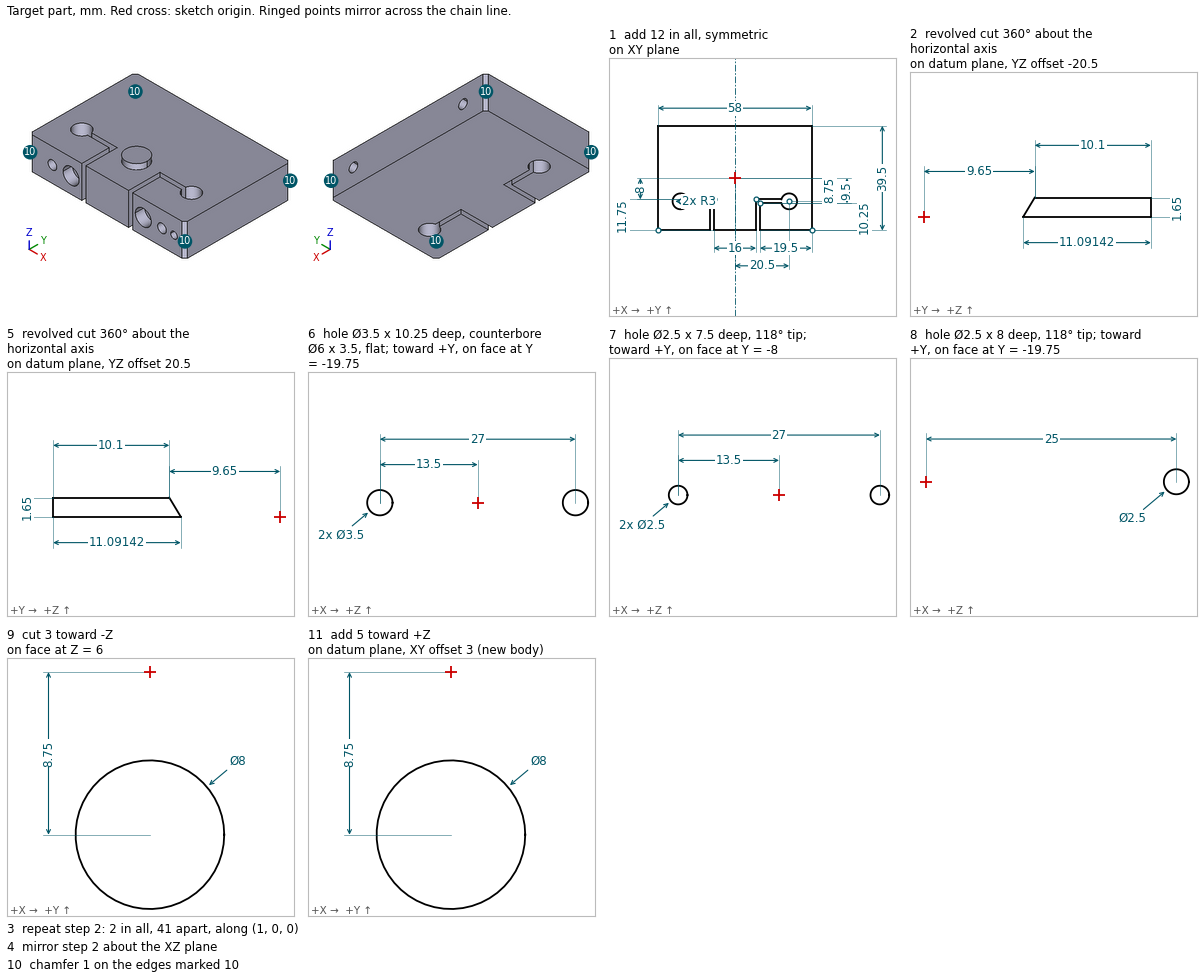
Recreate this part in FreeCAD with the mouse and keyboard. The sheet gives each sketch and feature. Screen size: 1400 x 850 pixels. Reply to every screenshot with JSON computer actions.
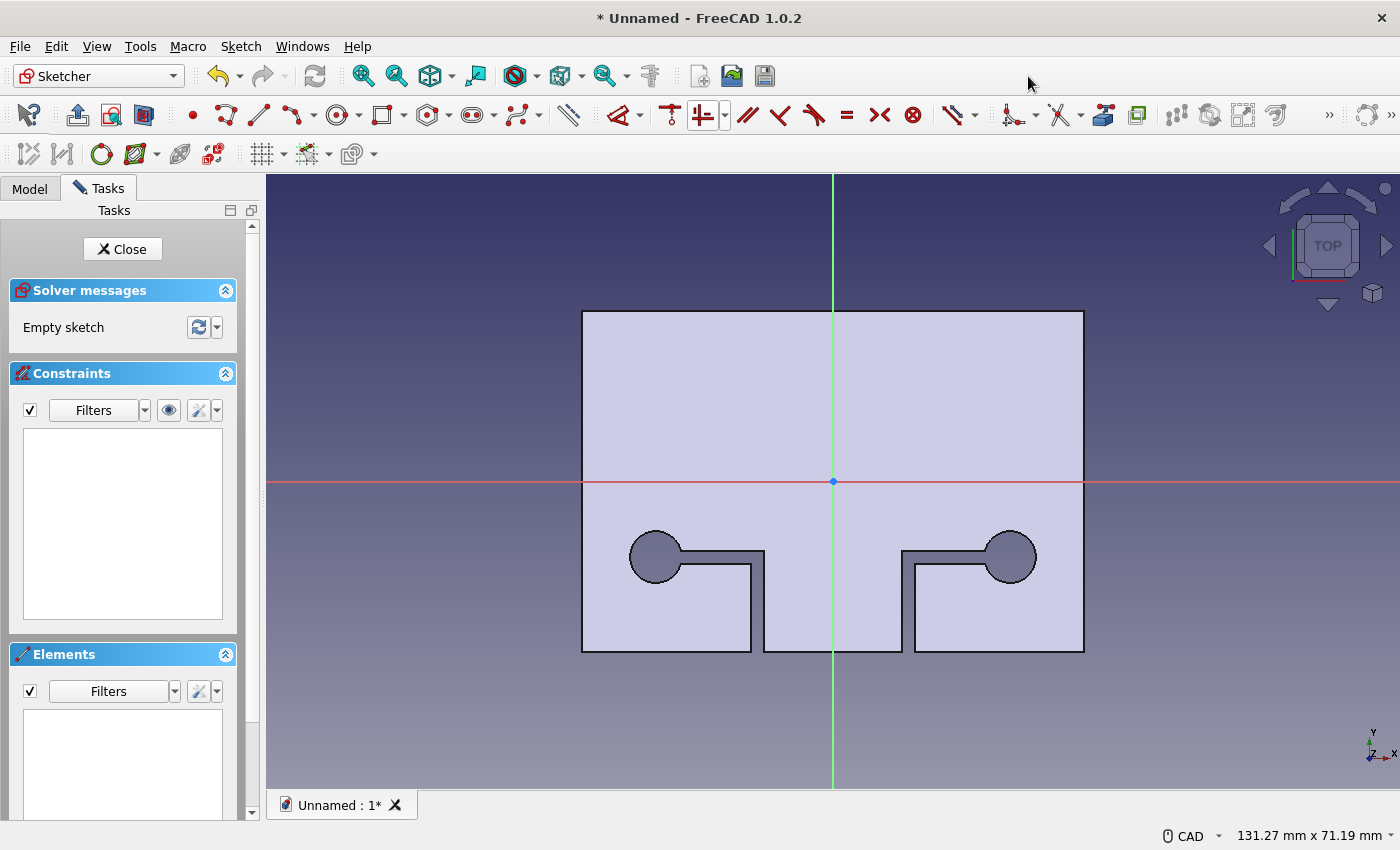
{"action": "scroll", "coordinate": [863, 560], "scroll_direction": "up", "scroll_amount": 6}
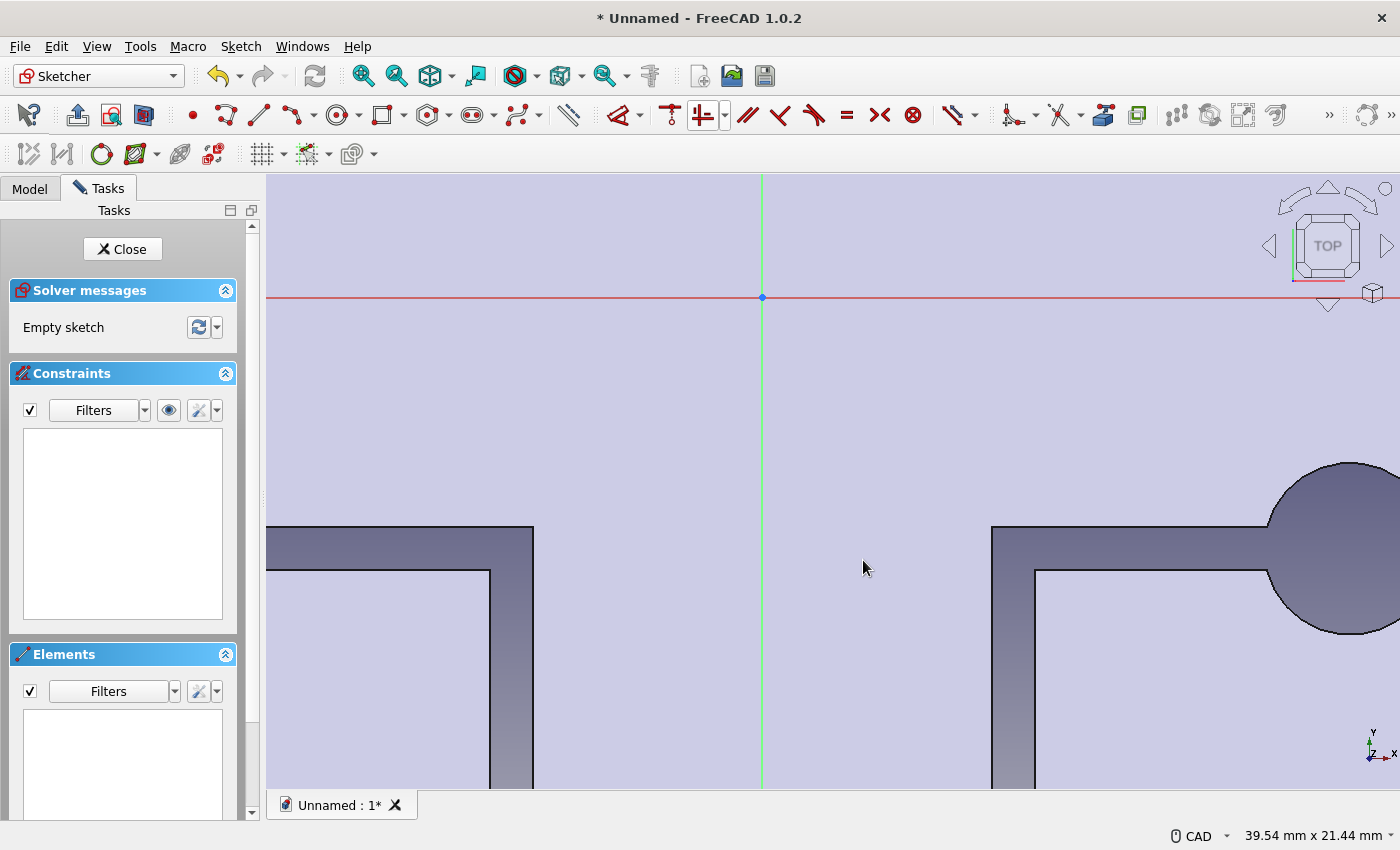
{"action": "left_click", "coordinate": [336, 116]}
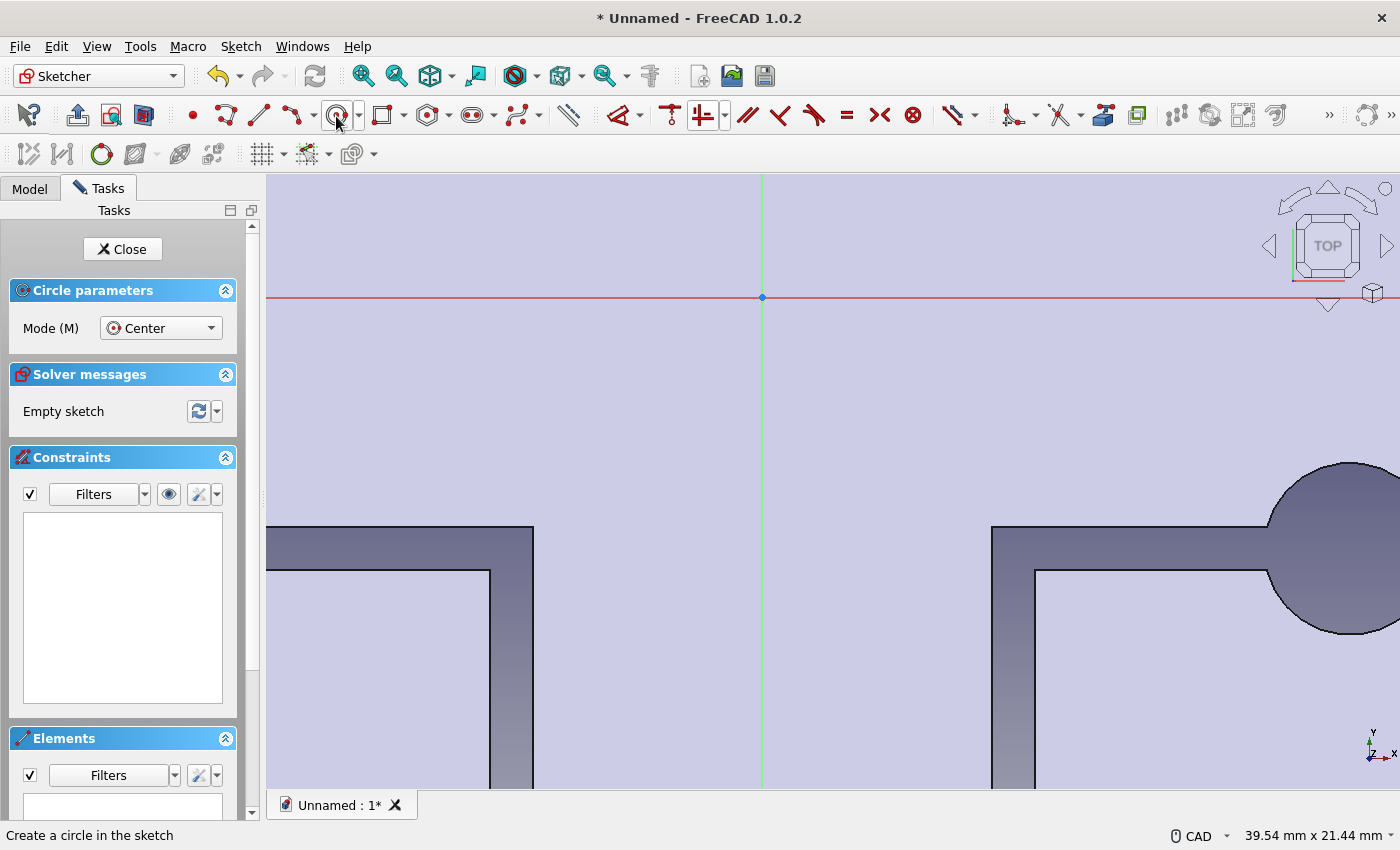
{"action": "left_click", "coordinate": [762, 549]}
{"action": "left_click", "coordinate": [843, 468]}
{"action": "key", "text": "Escape"}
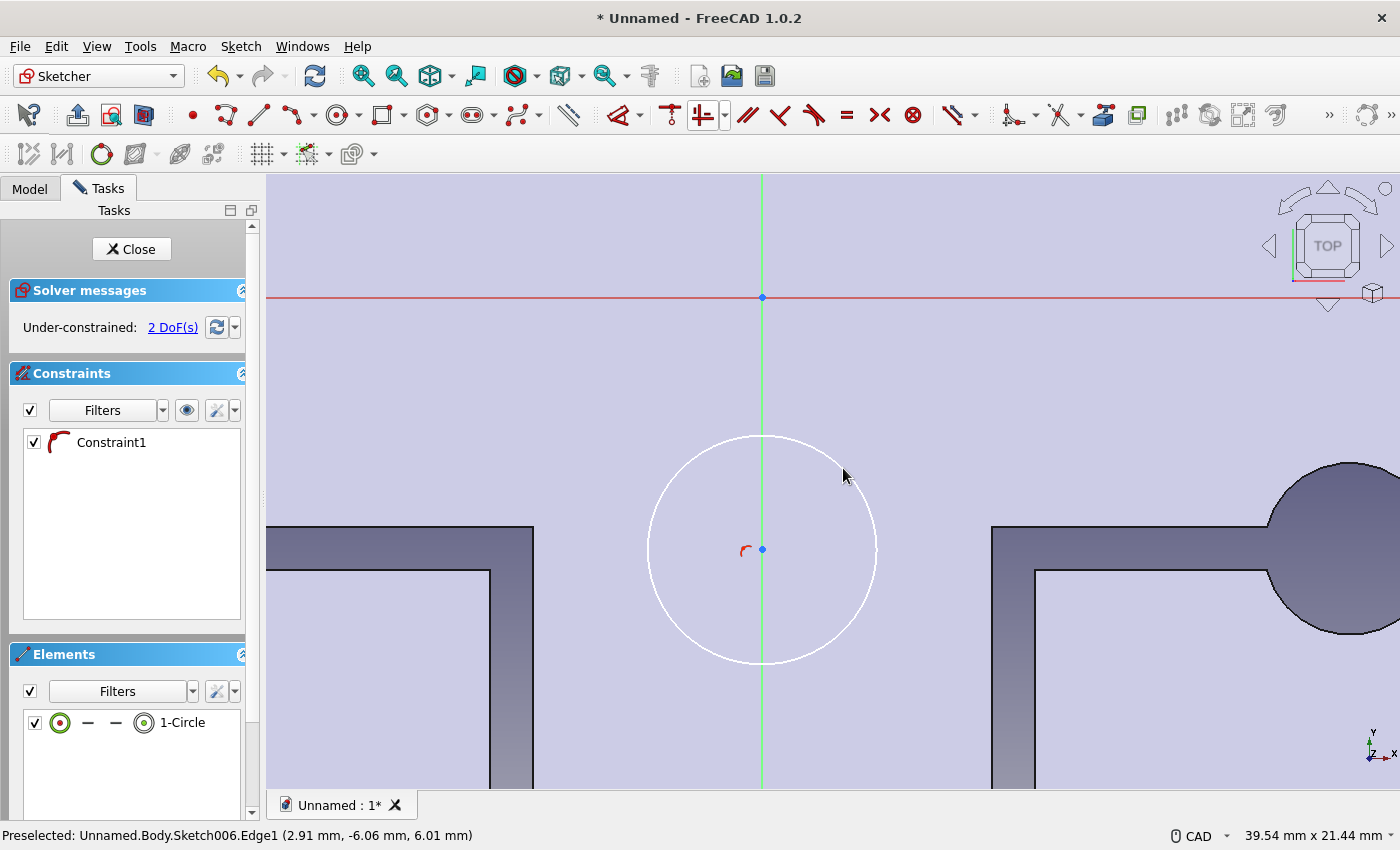
{"action": "key", "text": "d"}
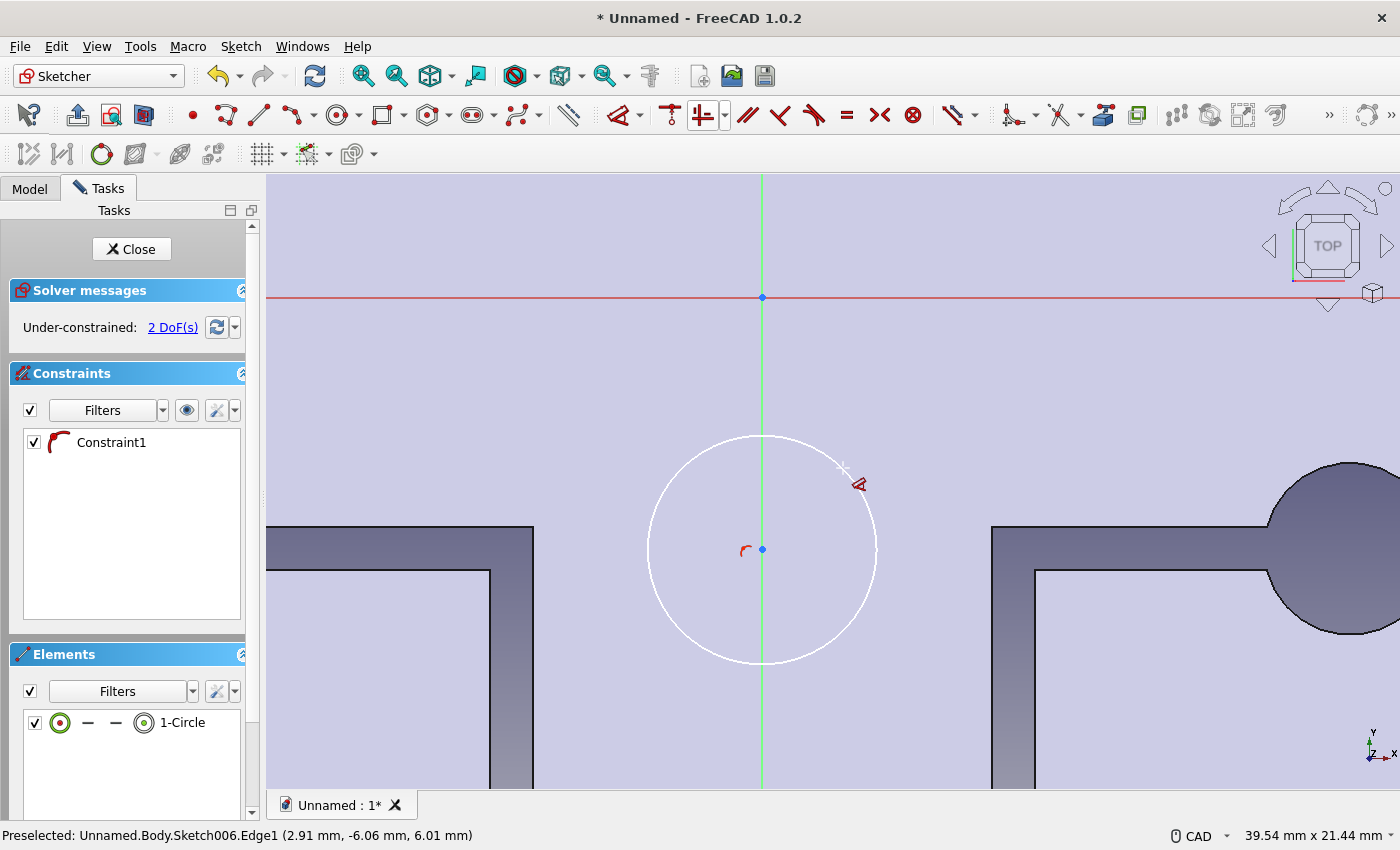
{"action": "left_click", "coordinate": [843, 469]}
{"action": "left_click", "coordinate": [866, 446]}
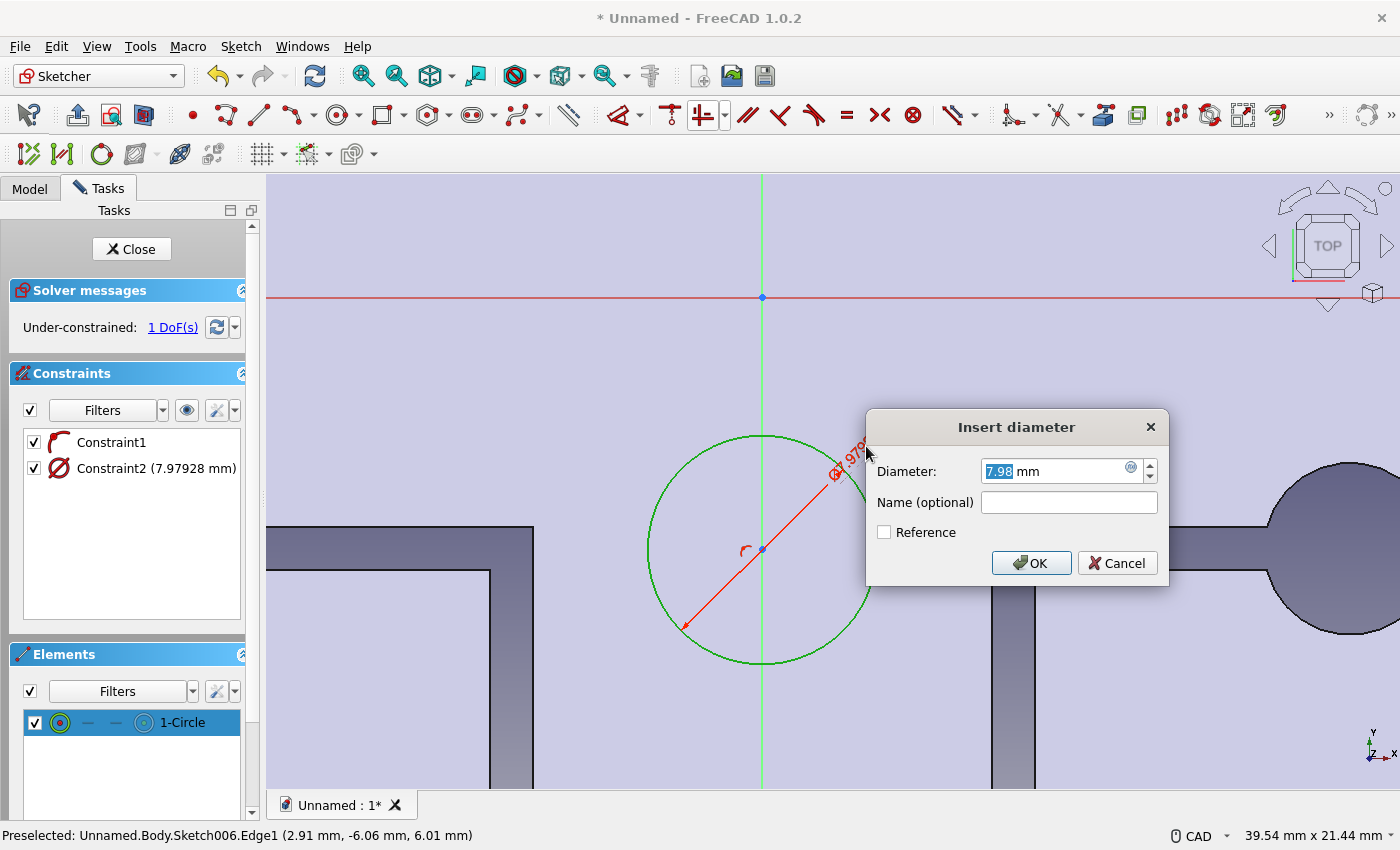
{"action": "type", "text": "8"}
{"action": "key", "text": "Return"}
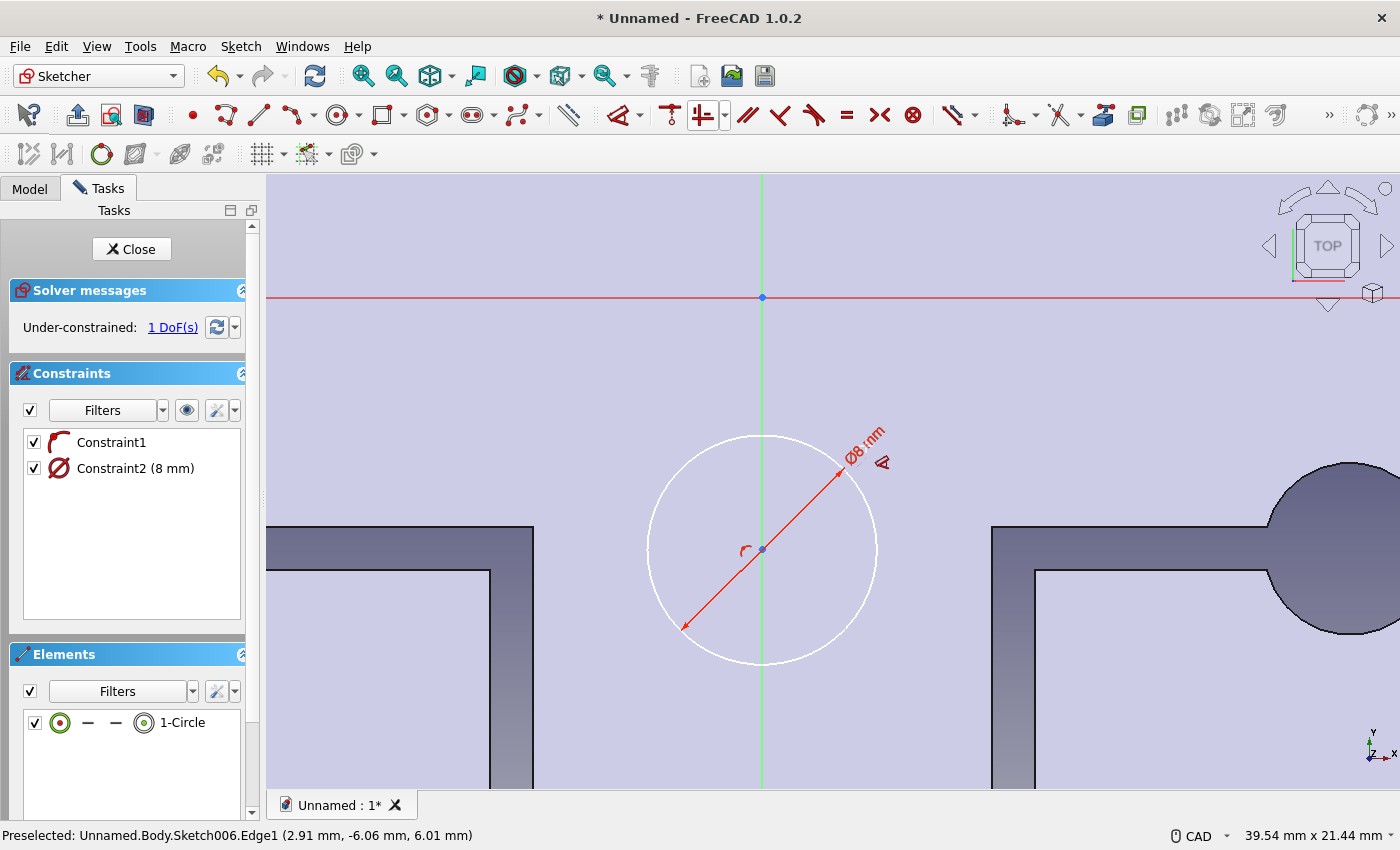
{"action": "left_click", "coordinate": [762, 550]}
{"action": "left_click", "coordinate": [796, 424]}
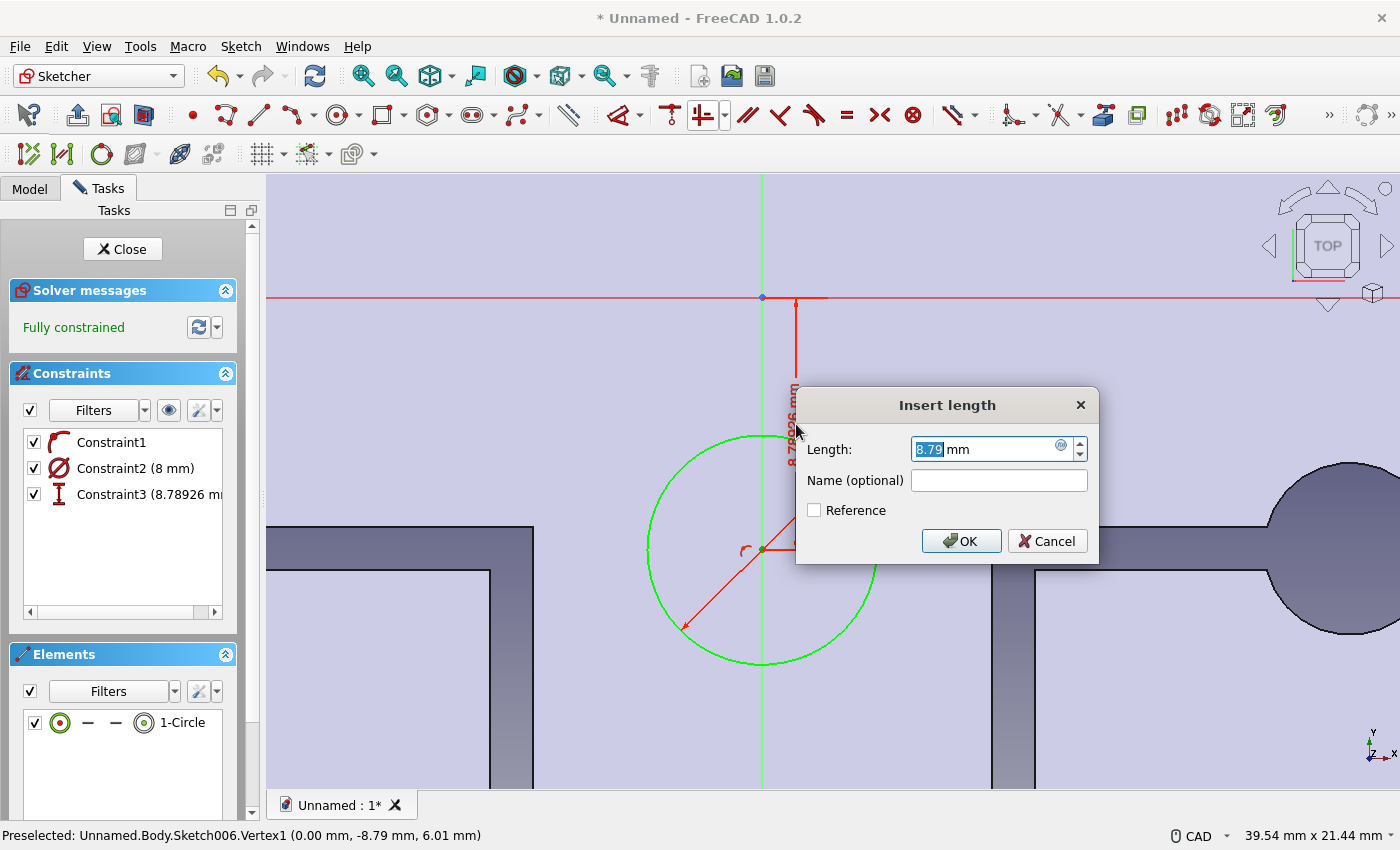
{"action": "type", "text": "8.75"}
{"action": "key", "text": "Return"}
{"action": "key", "text": "Escape"}